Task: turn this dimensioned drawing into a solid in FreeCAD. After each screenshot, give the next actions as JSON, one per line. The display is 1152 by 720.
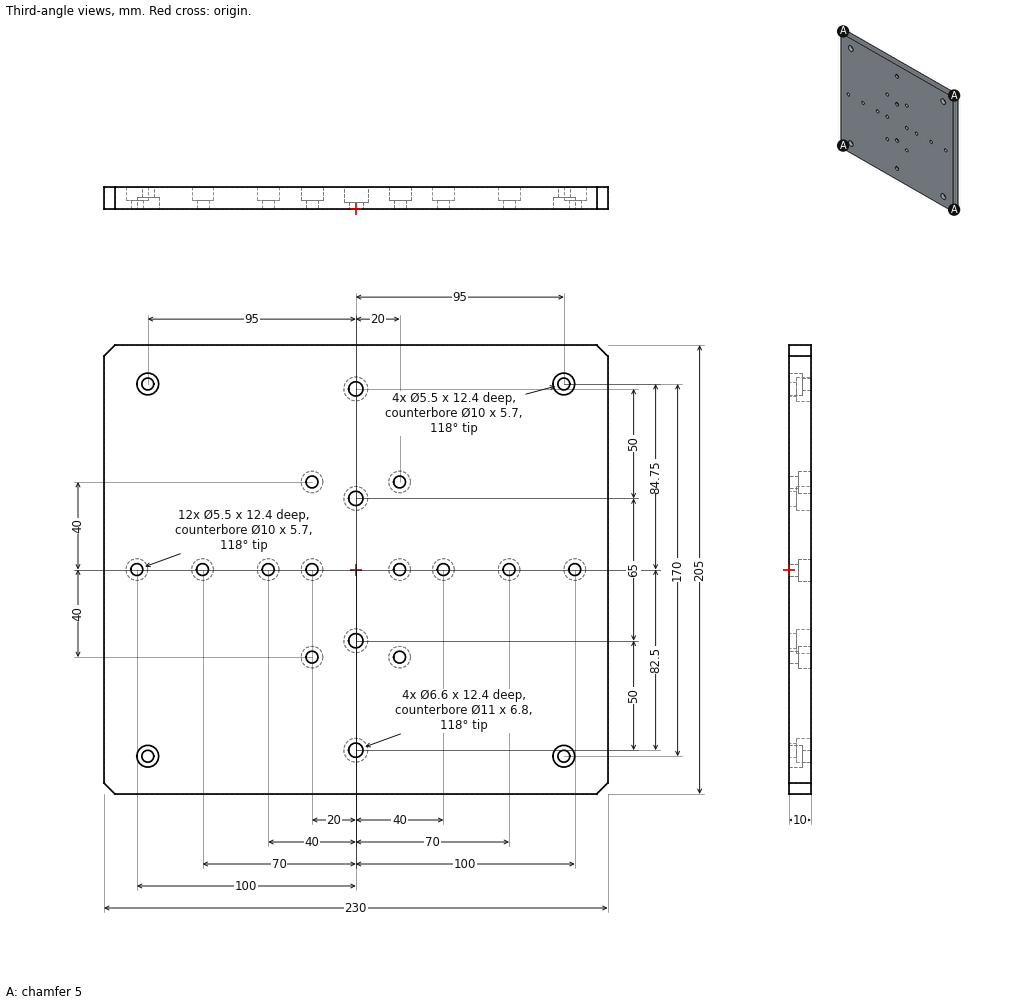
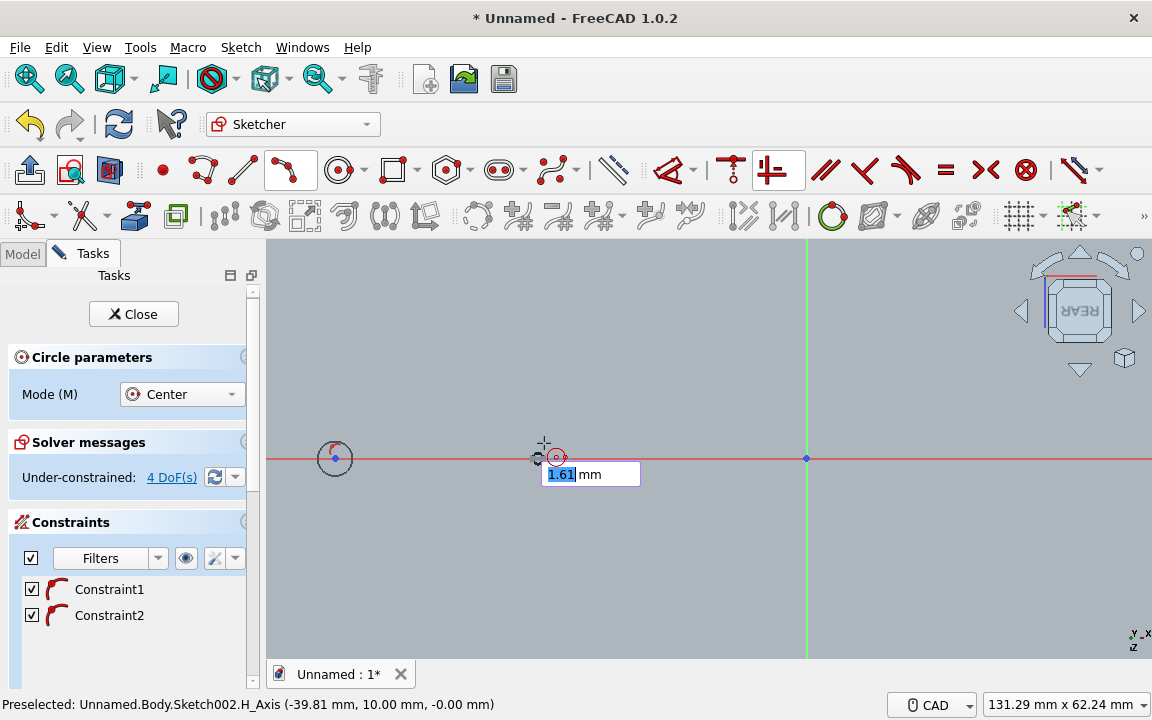
{"action": "left_click", "coordinate": [543, 441]}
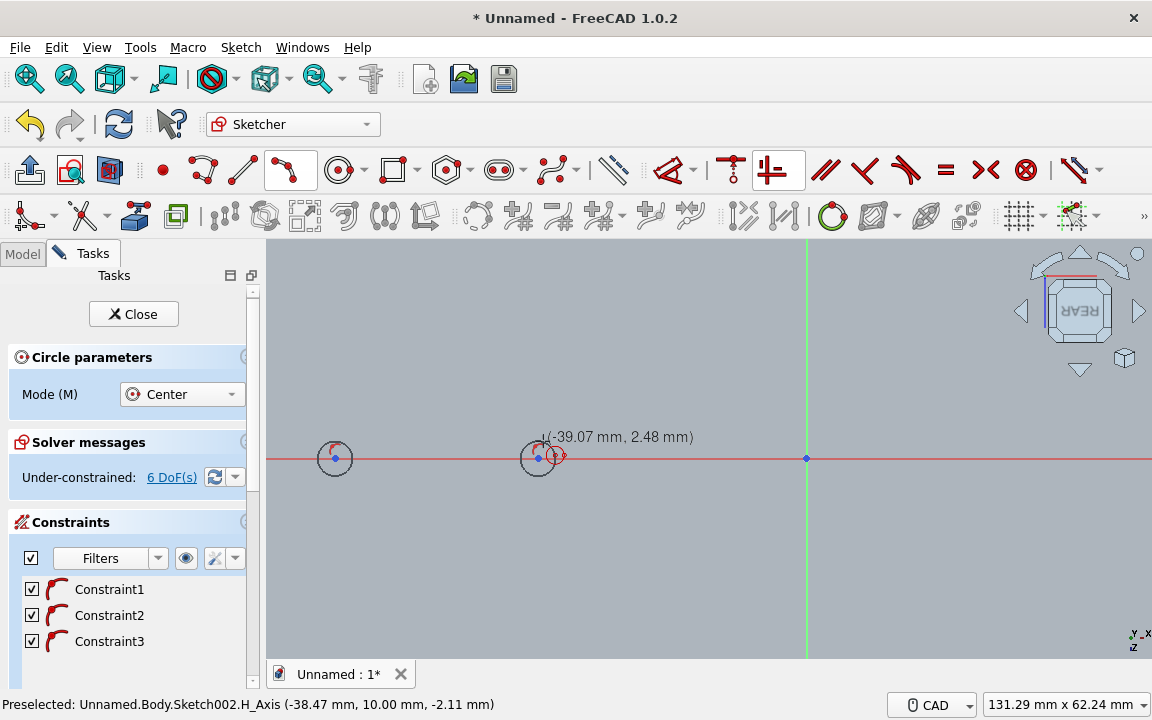
{"action": "scroll", "coordinate": [672, 459], "scroll_direction": "up", "scroll_amount": 2}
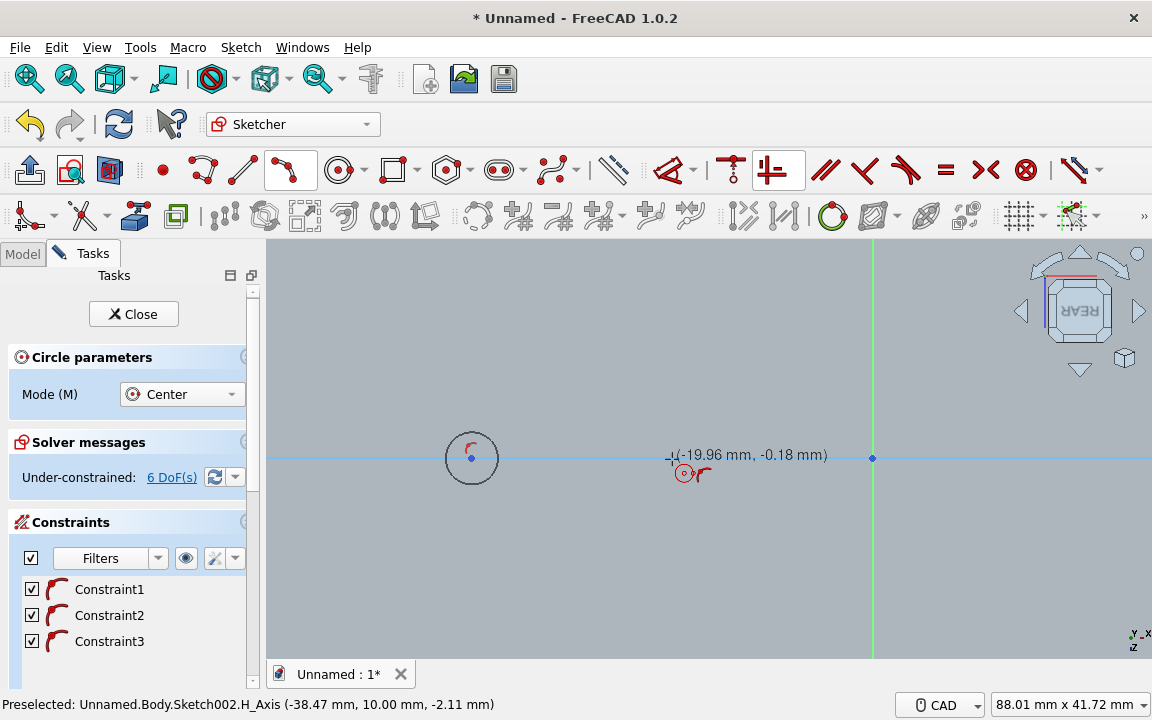
{"action": "scroll", "coordinate": [565, 446], "scroll_direction": "down", "scroll_amount": 7}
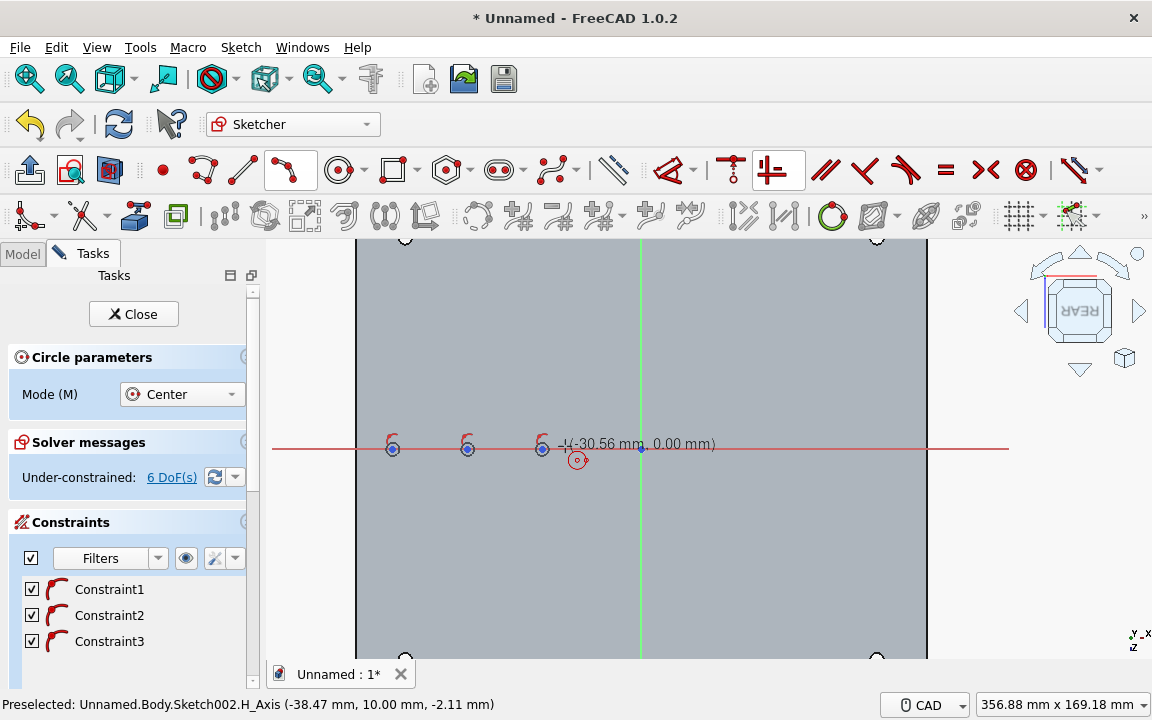
{"action": "left_click", "coordinate": [591, 449]}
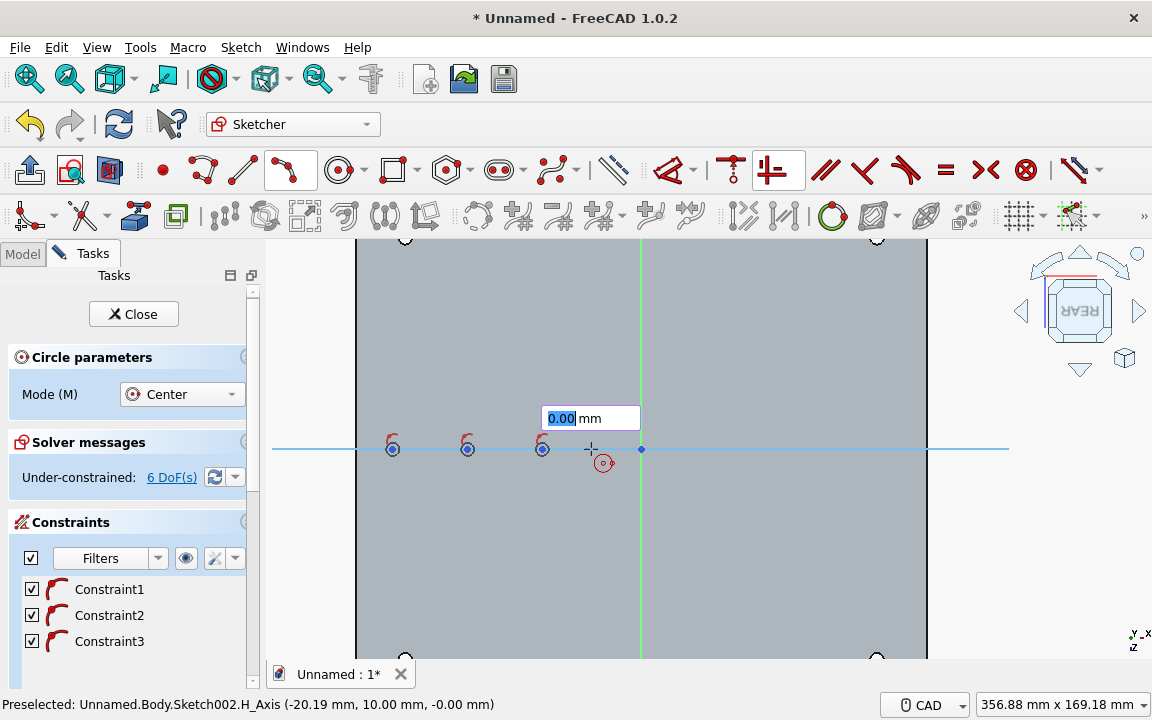
{"action": "scroll", "coordinate": [594, 443], "scroll_direction": "up", "scroll_amount": 5}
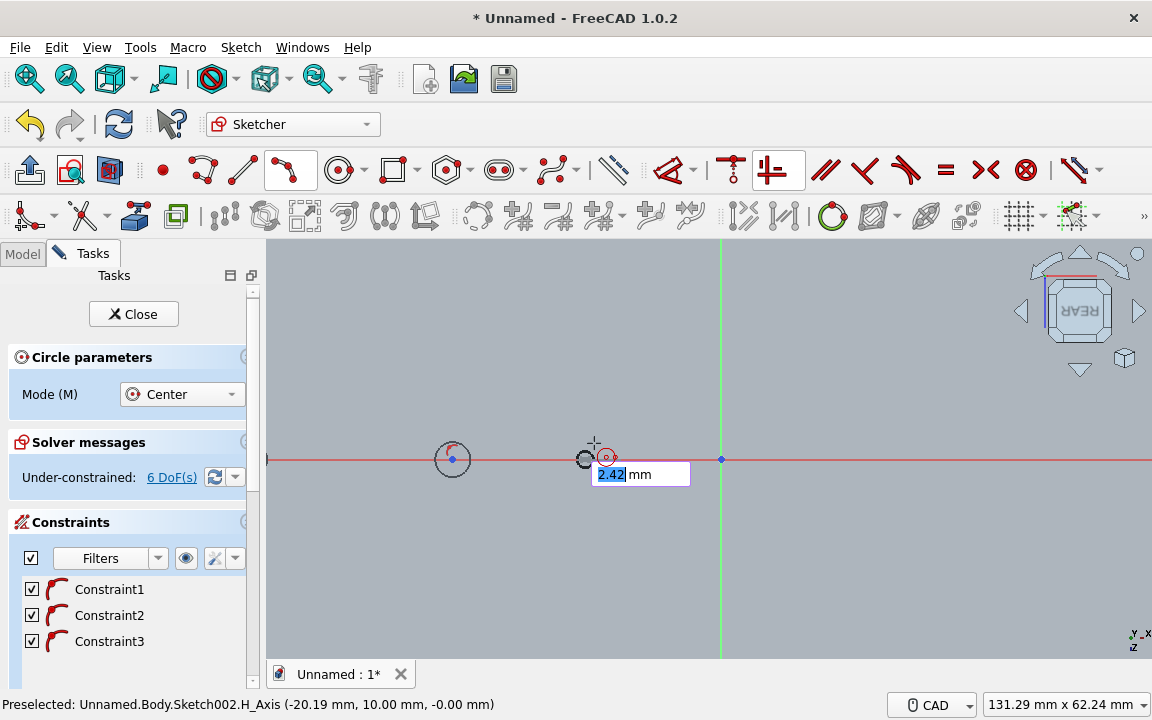
{"action": "left_click", "coordinate": [593, 442]}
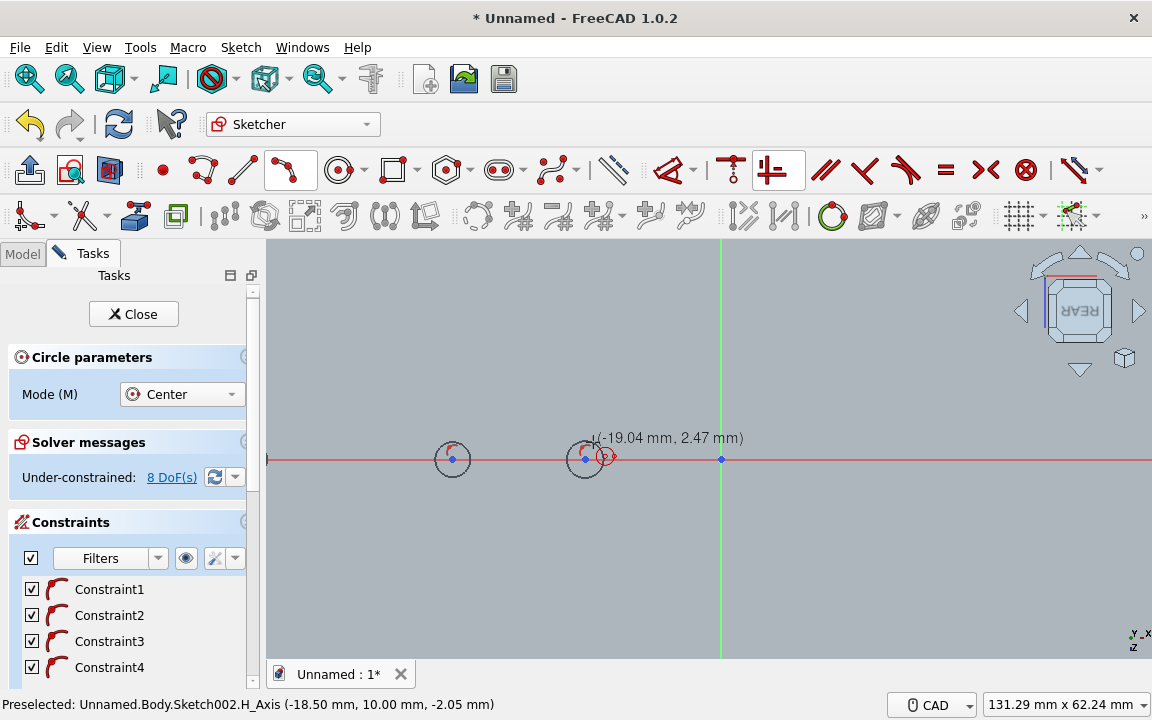
{"action": "scroll", "coordinate": [593, 443], "scroll_direction": "down", "scroll_amount": 5}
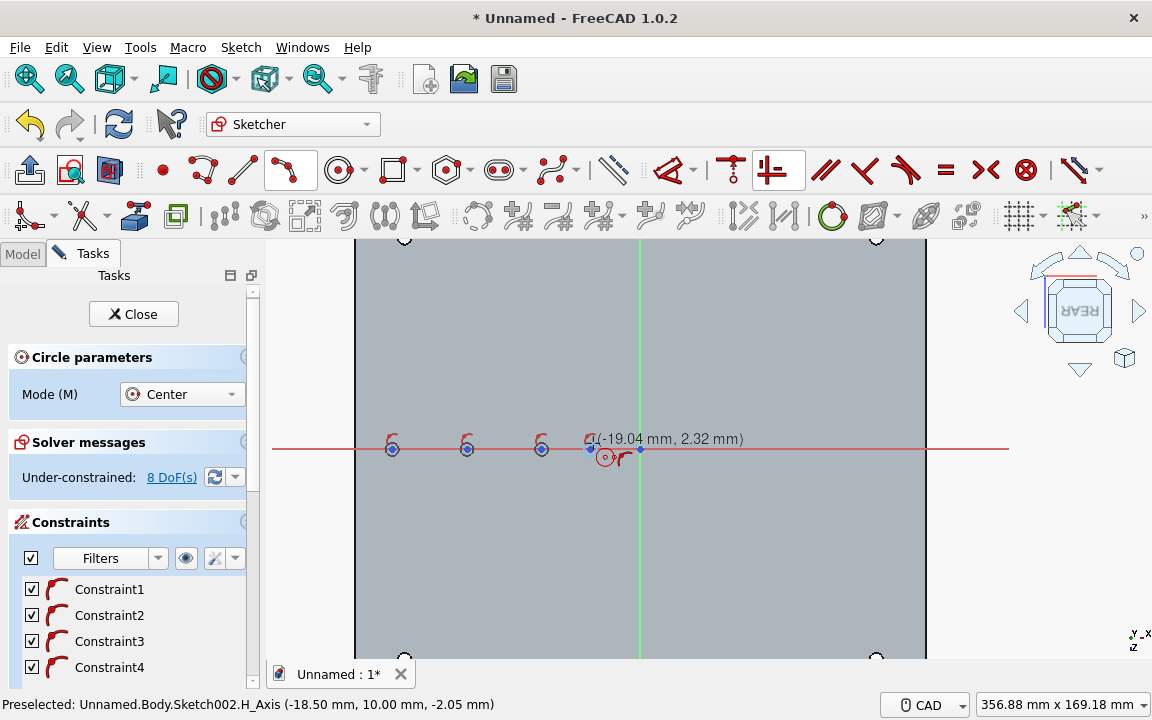
{"action": "scroll", "coordinate": [591, 350], "scroll_direction": "up", "scroll_amount": 7}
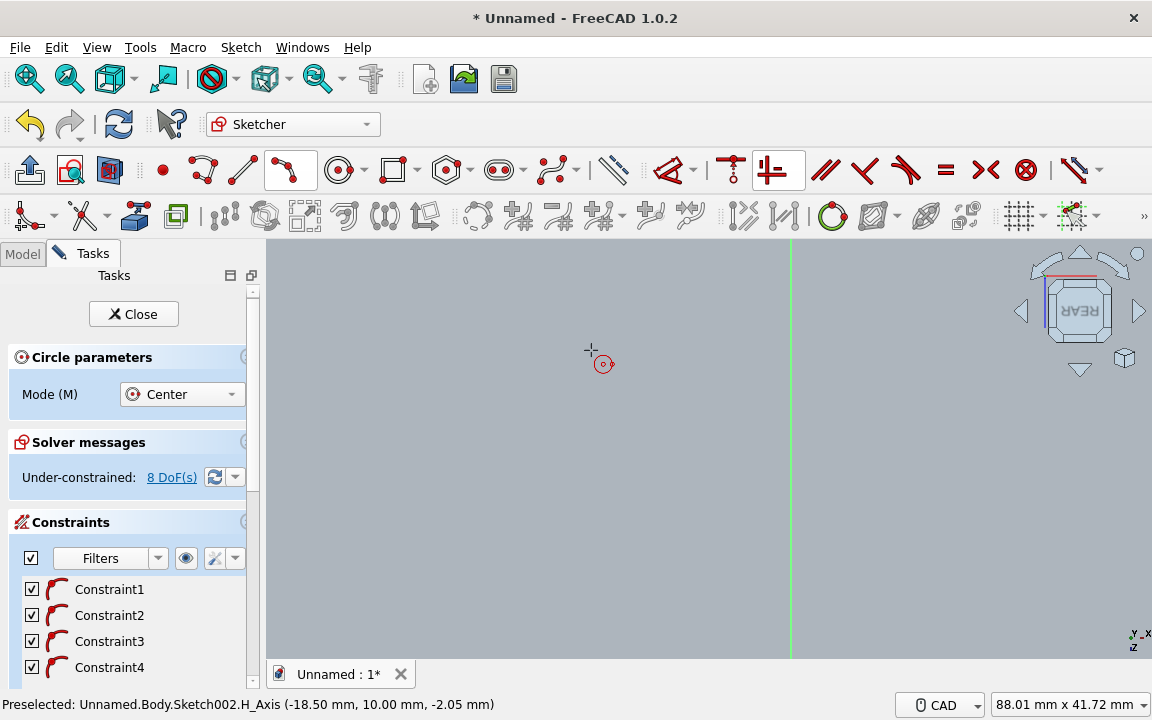
{"action": "scroll", "coordinate": [591, 350], "scroll_direction": "down", "scroll_amount": 7}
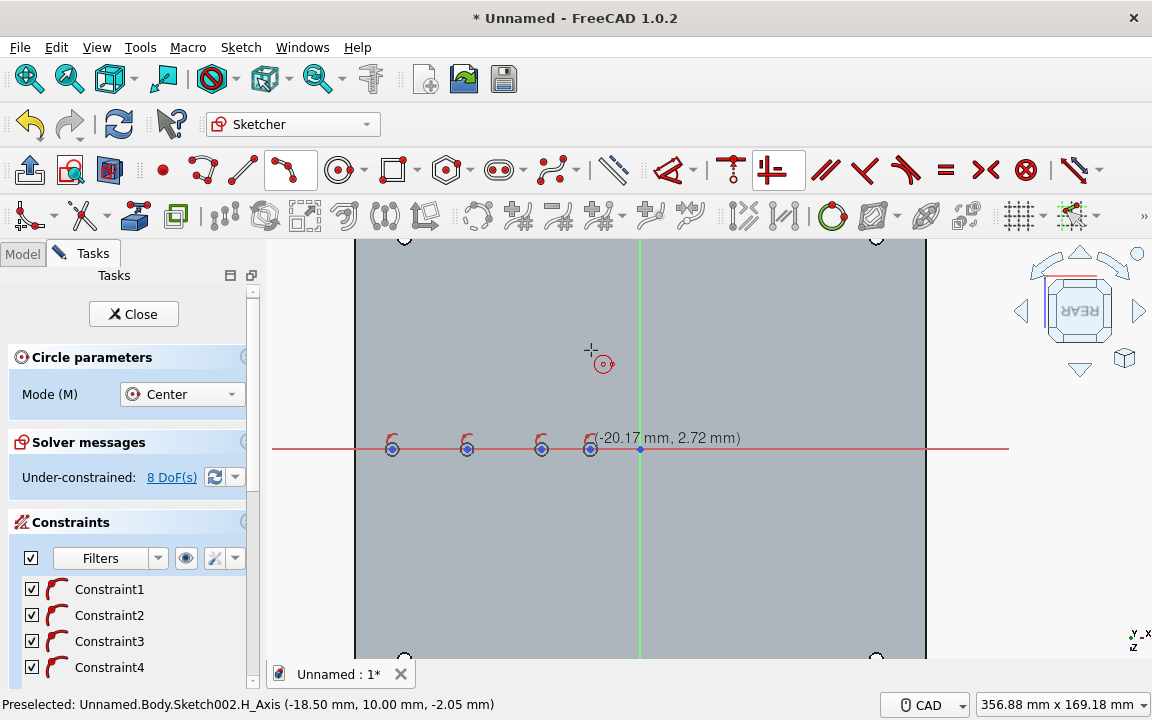
{"action": "left_click", "coordinate": [591, 350]}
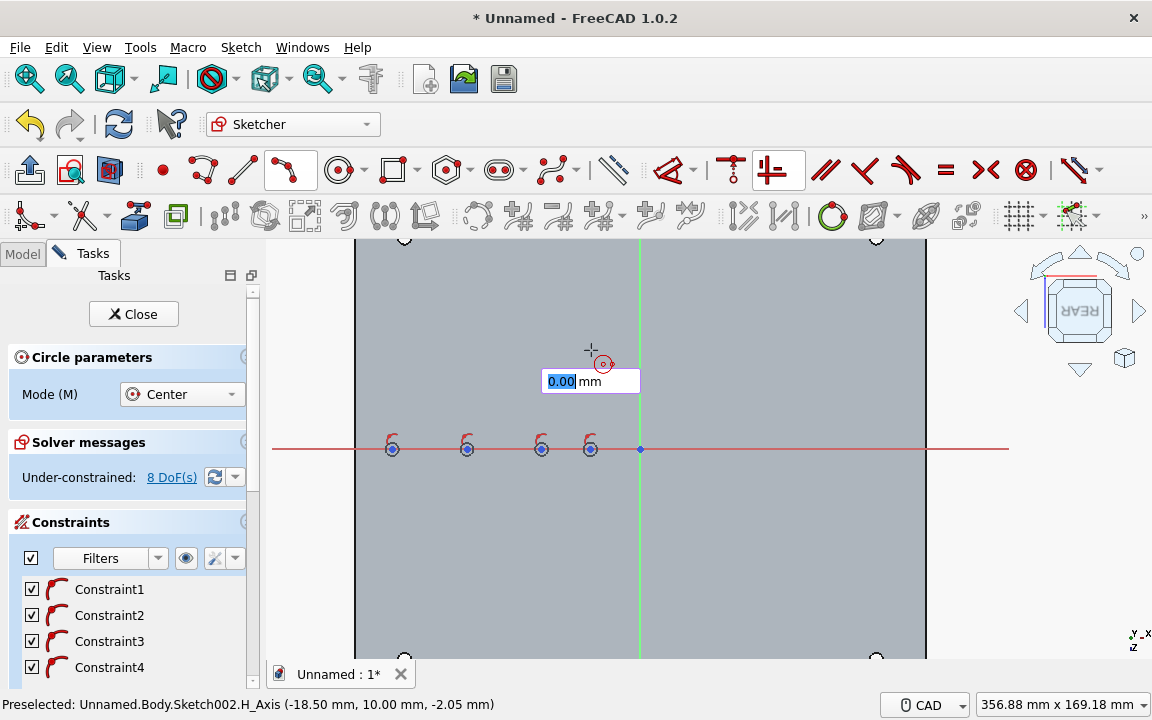
{"action": "scroll", "coordinate": [596, 345], "scroll_direction": "up", "scroll_amount": 5}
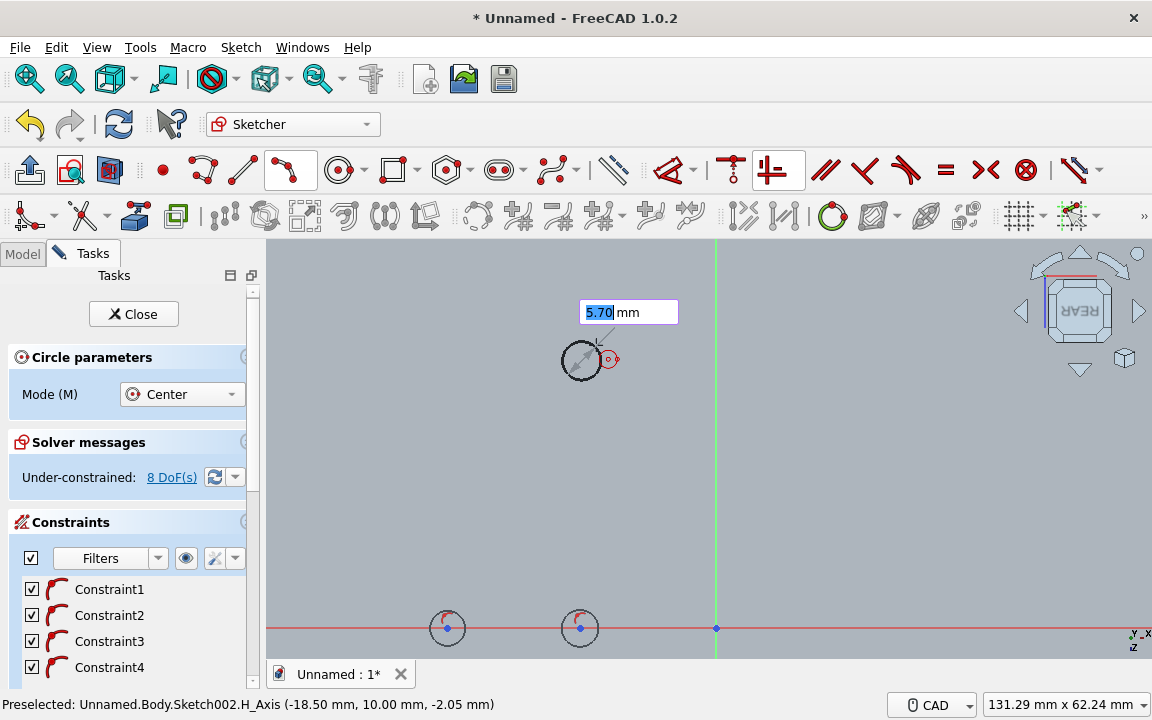
{"action": "left_click", "coordinate": [594, 345]}